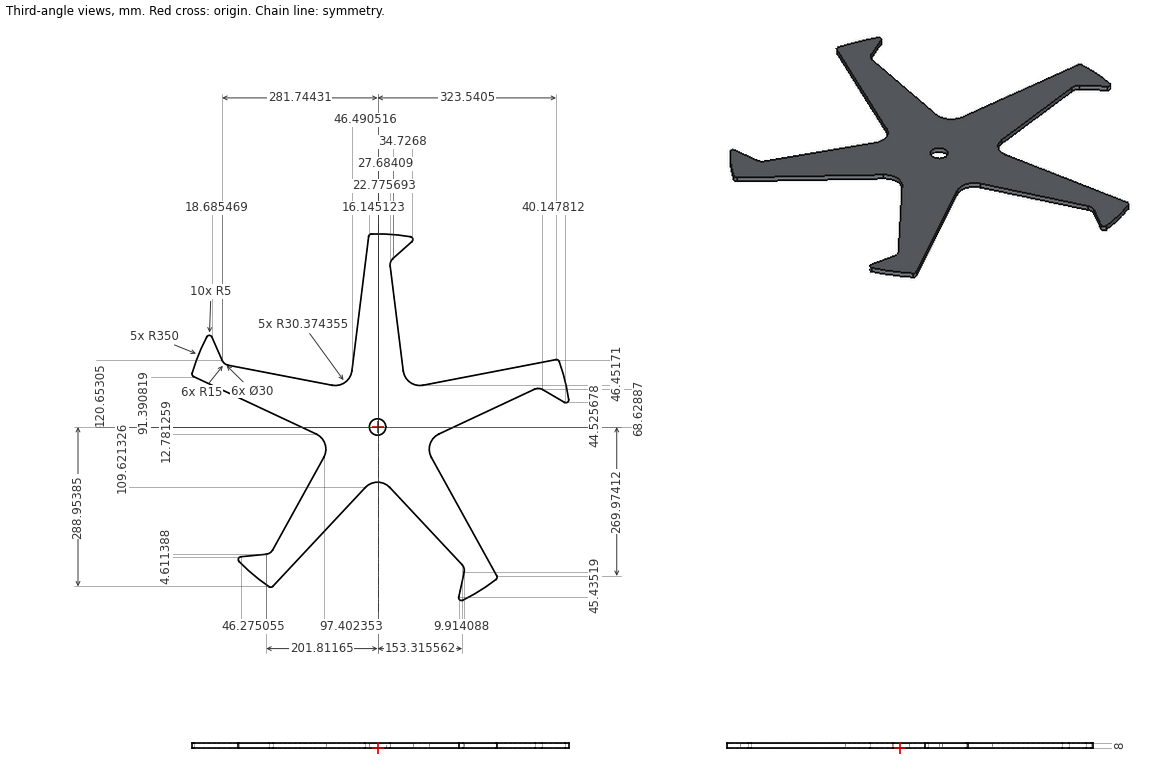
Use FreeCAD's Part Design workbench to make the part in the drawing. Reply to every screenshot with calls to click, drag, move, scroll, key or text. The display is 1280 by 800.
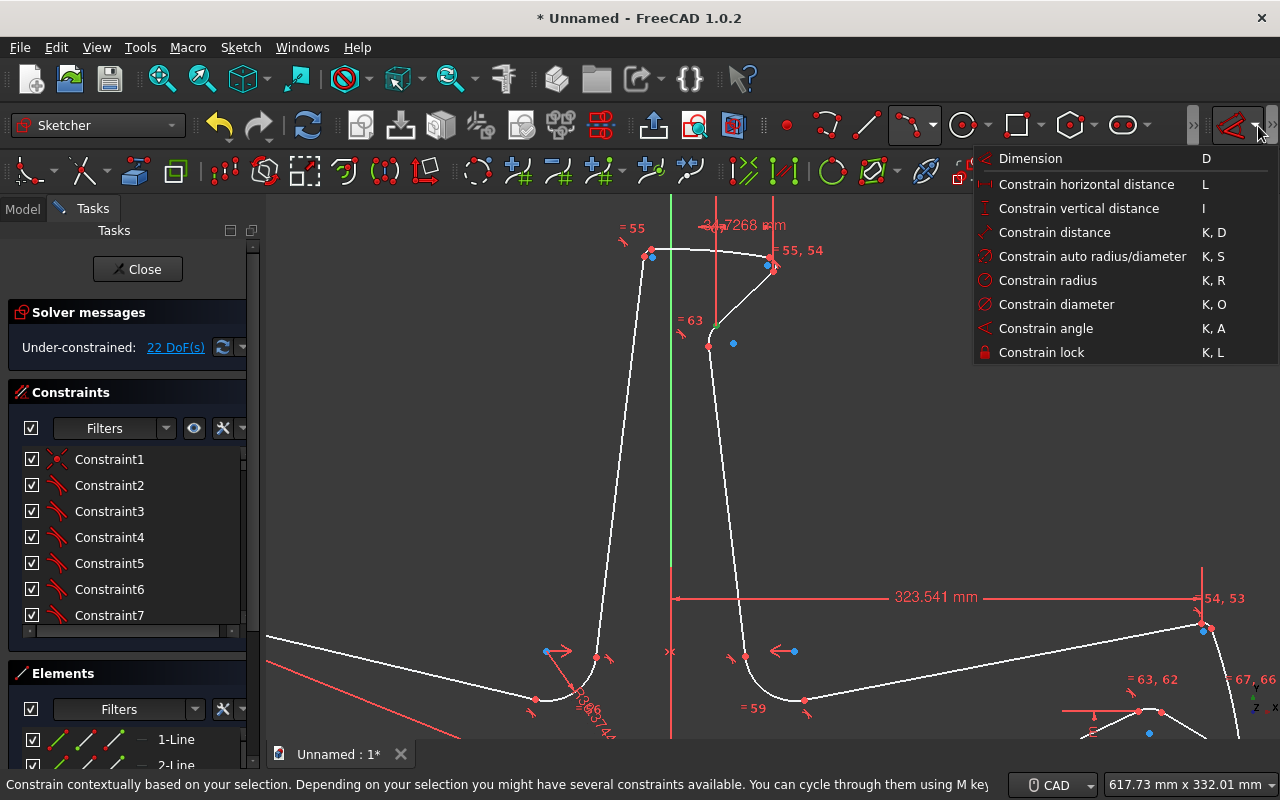
click(1126, 184)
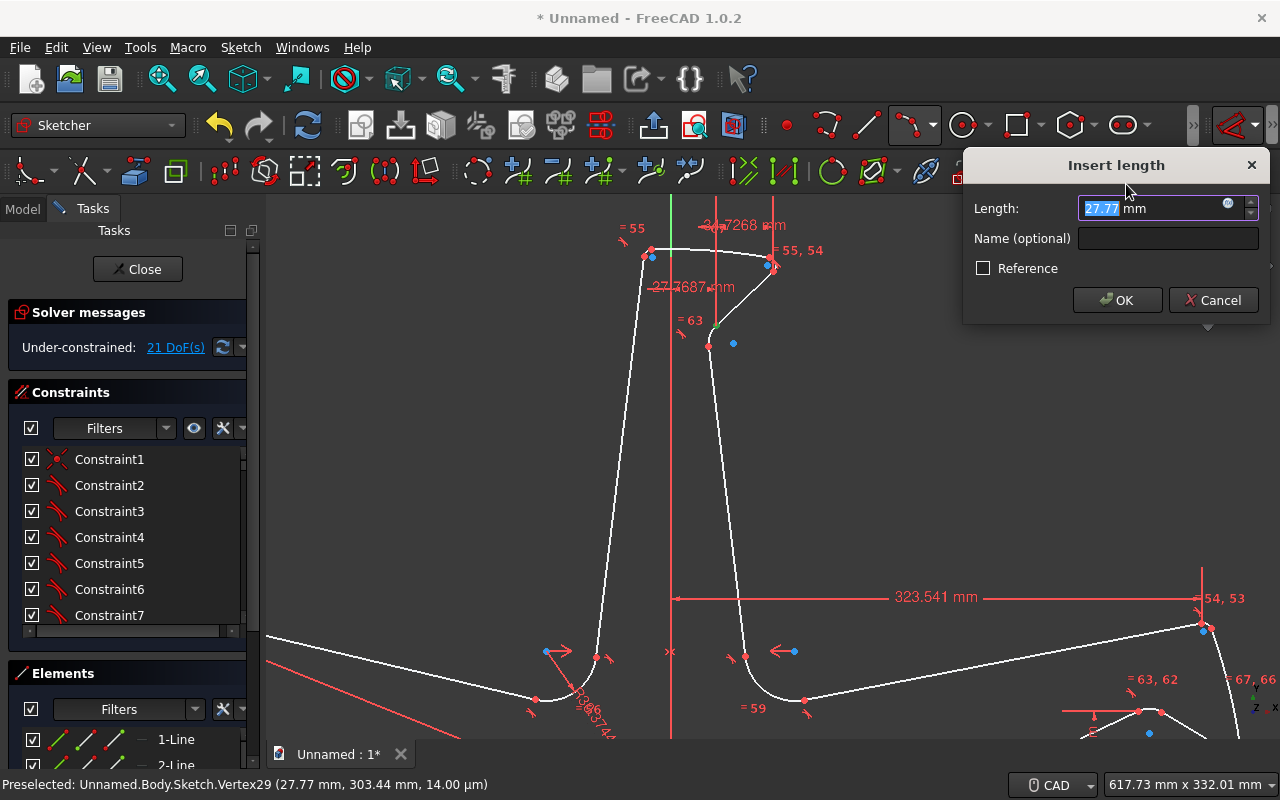
text(27.68409)
key(Return)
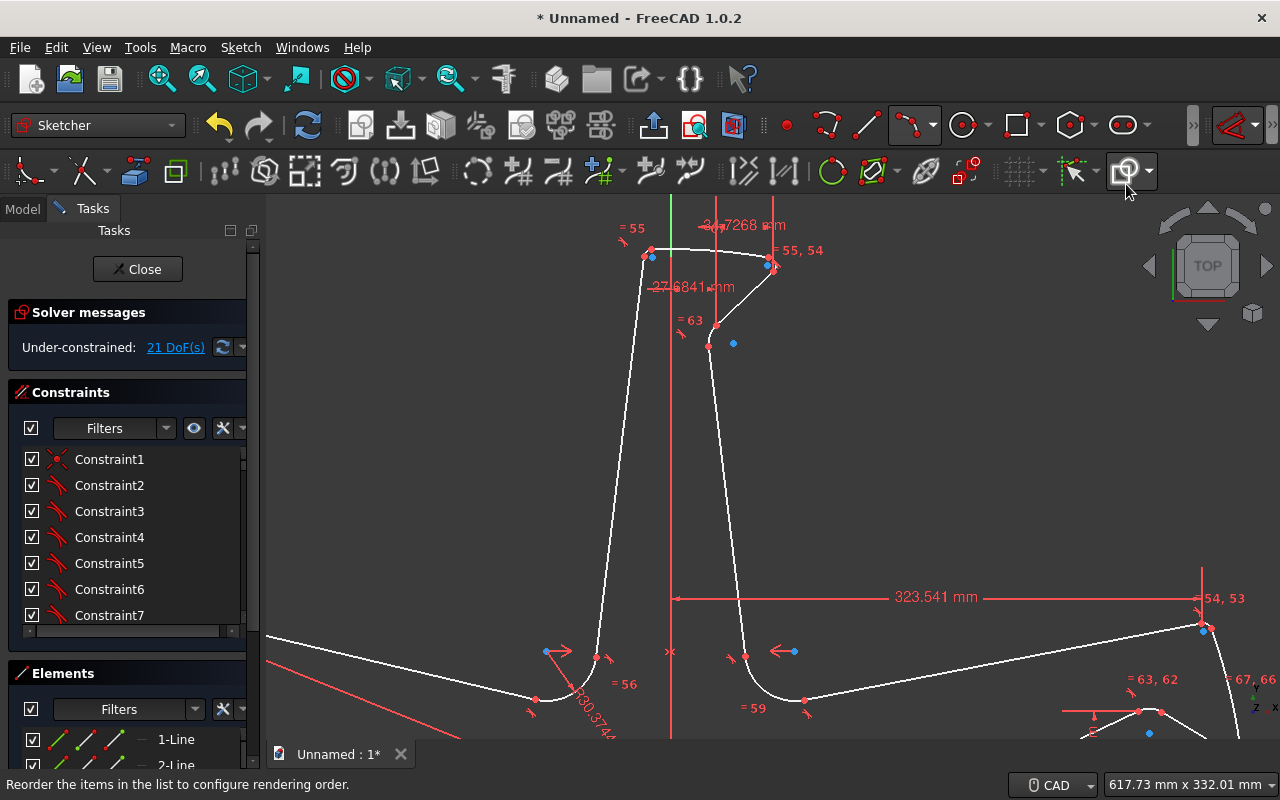
scroll(715, 325, down, 6)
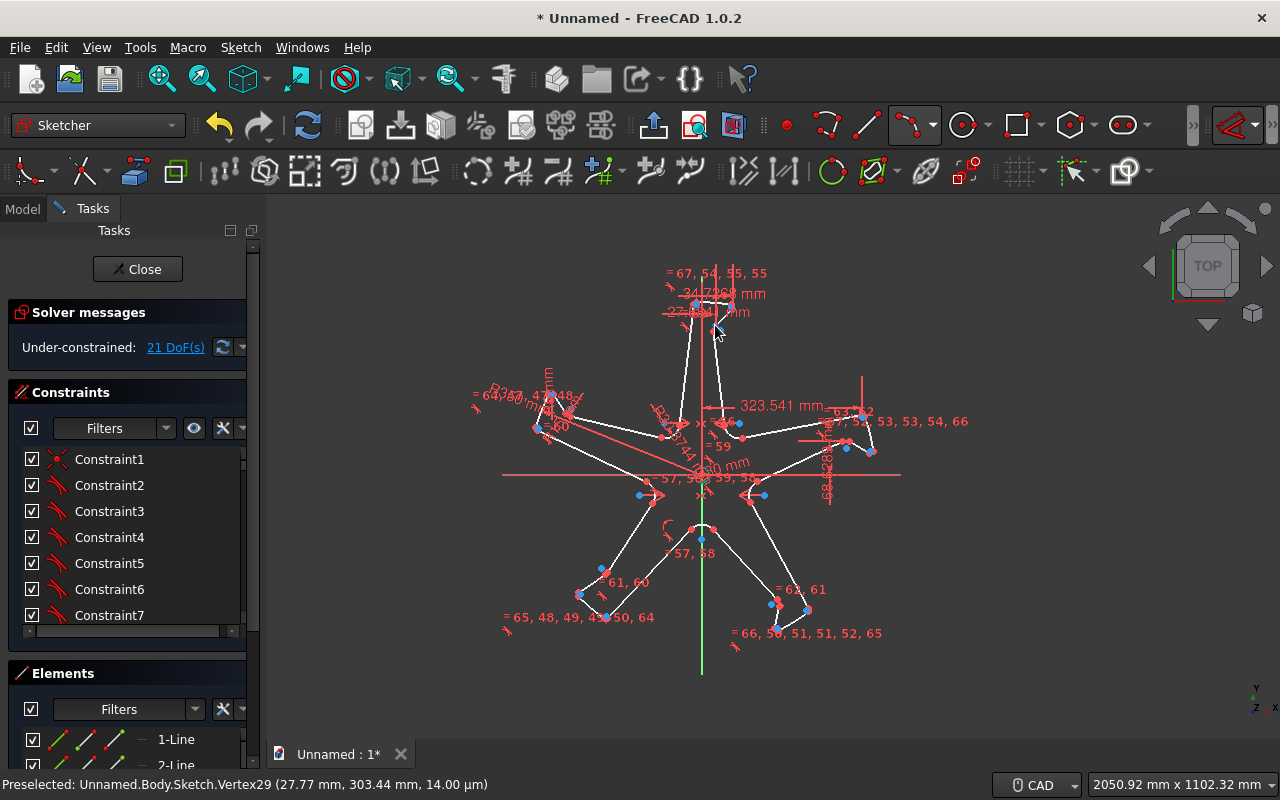
scroll(597, 580, up, 15)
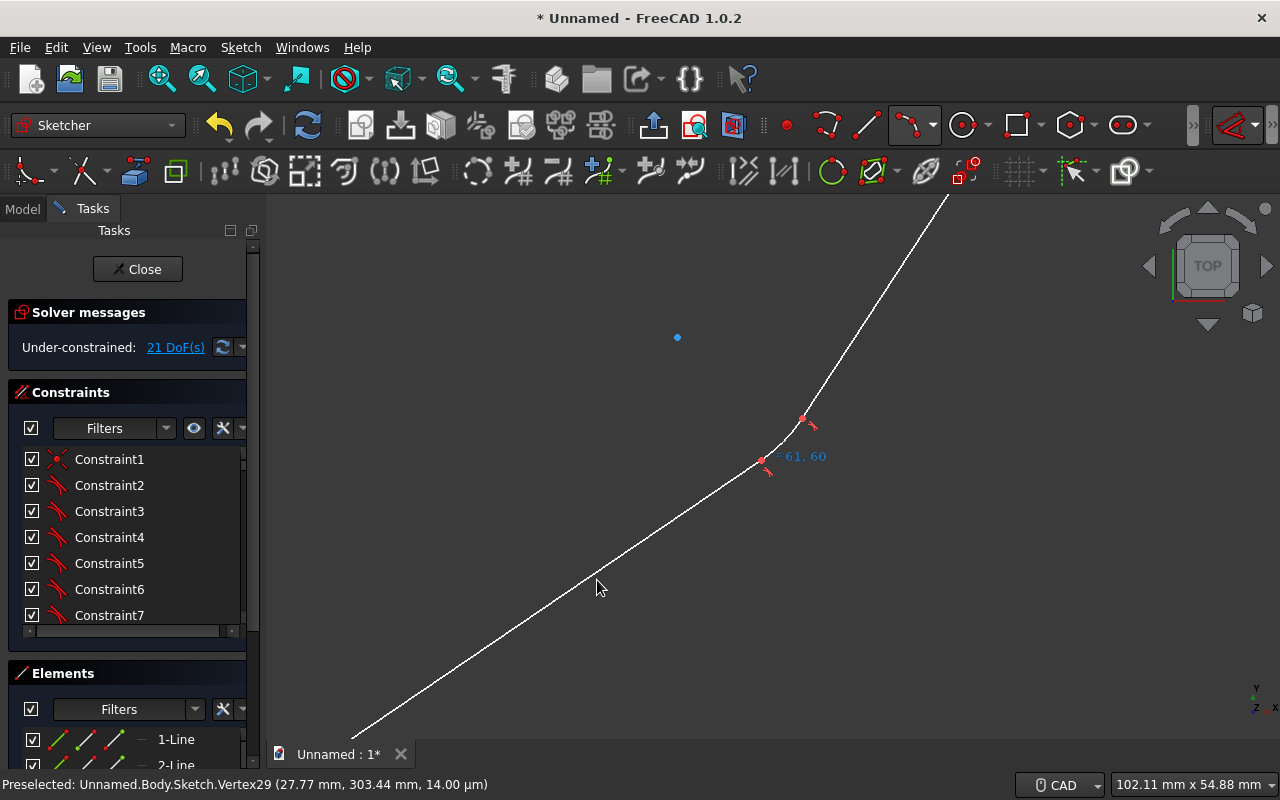
click(601, 569)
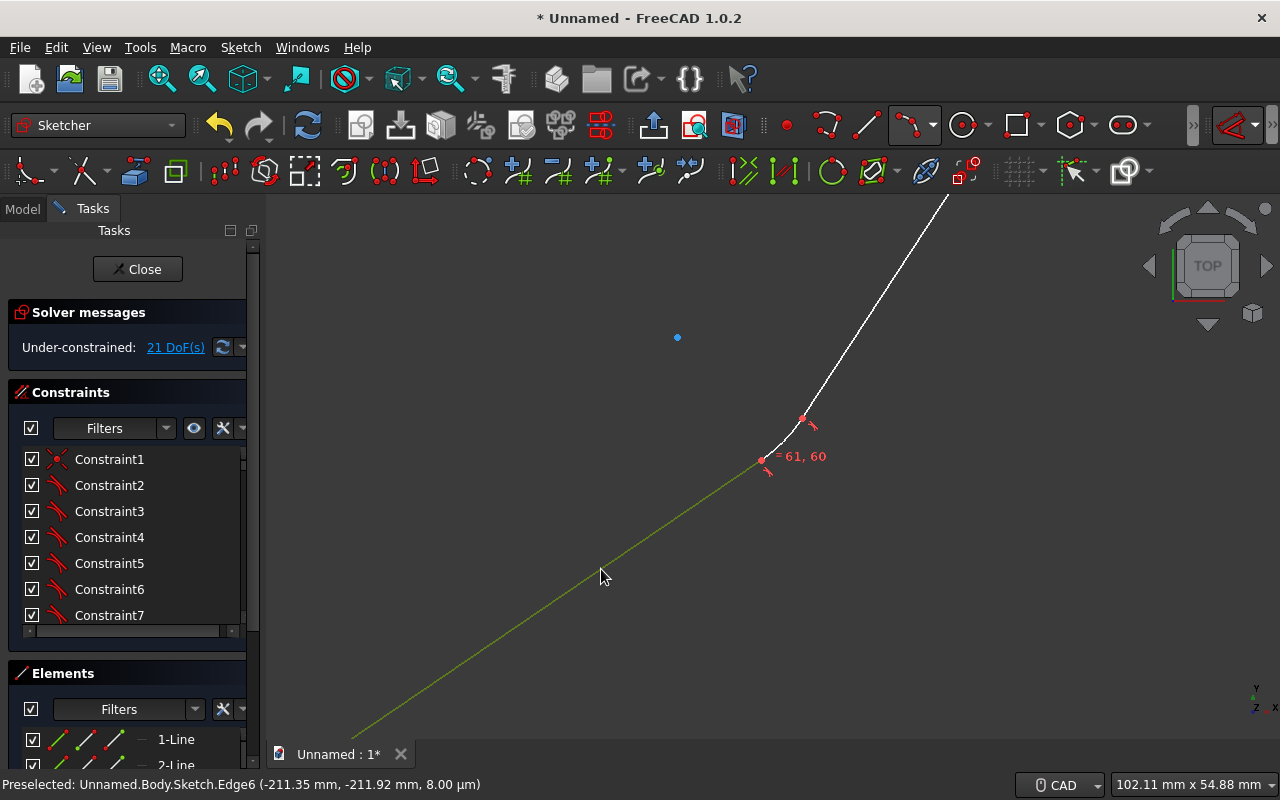
key(i)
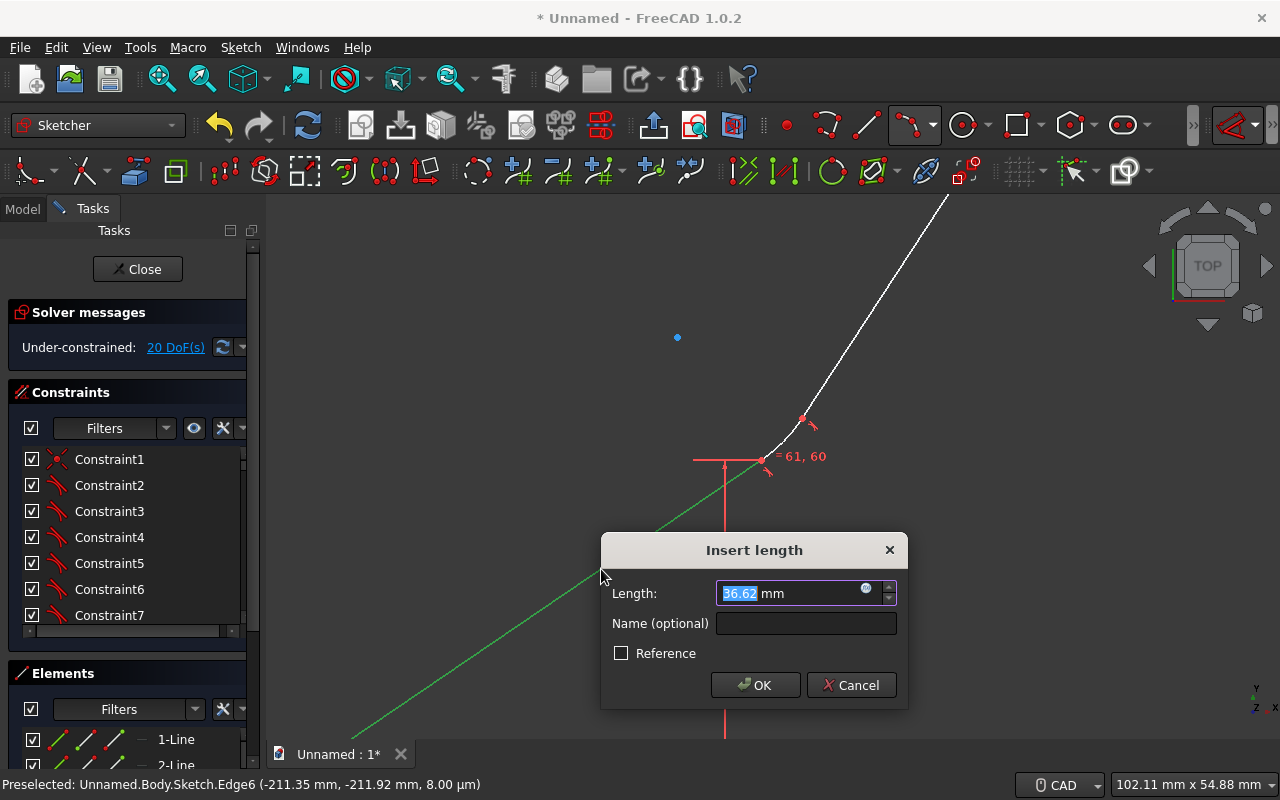
text(4.611388)
key(Return)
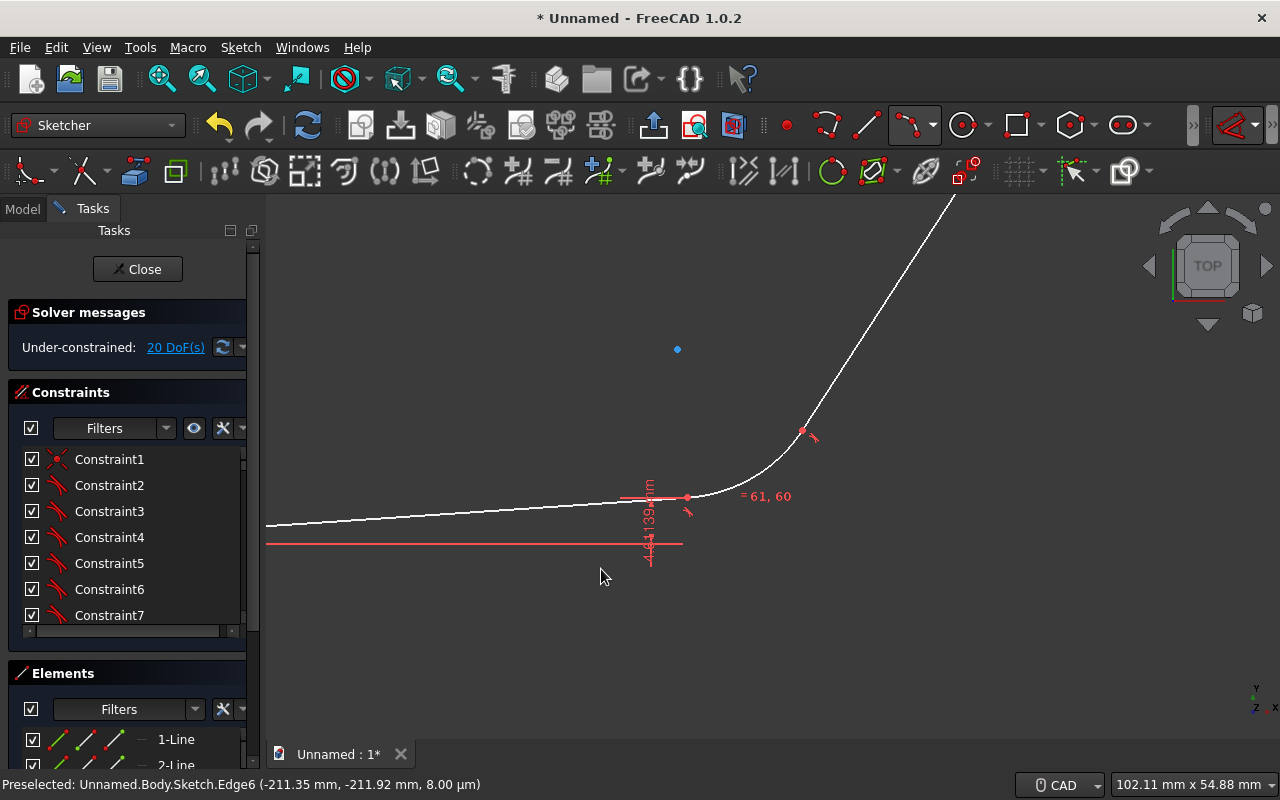
scroll(597, 581, down, 15)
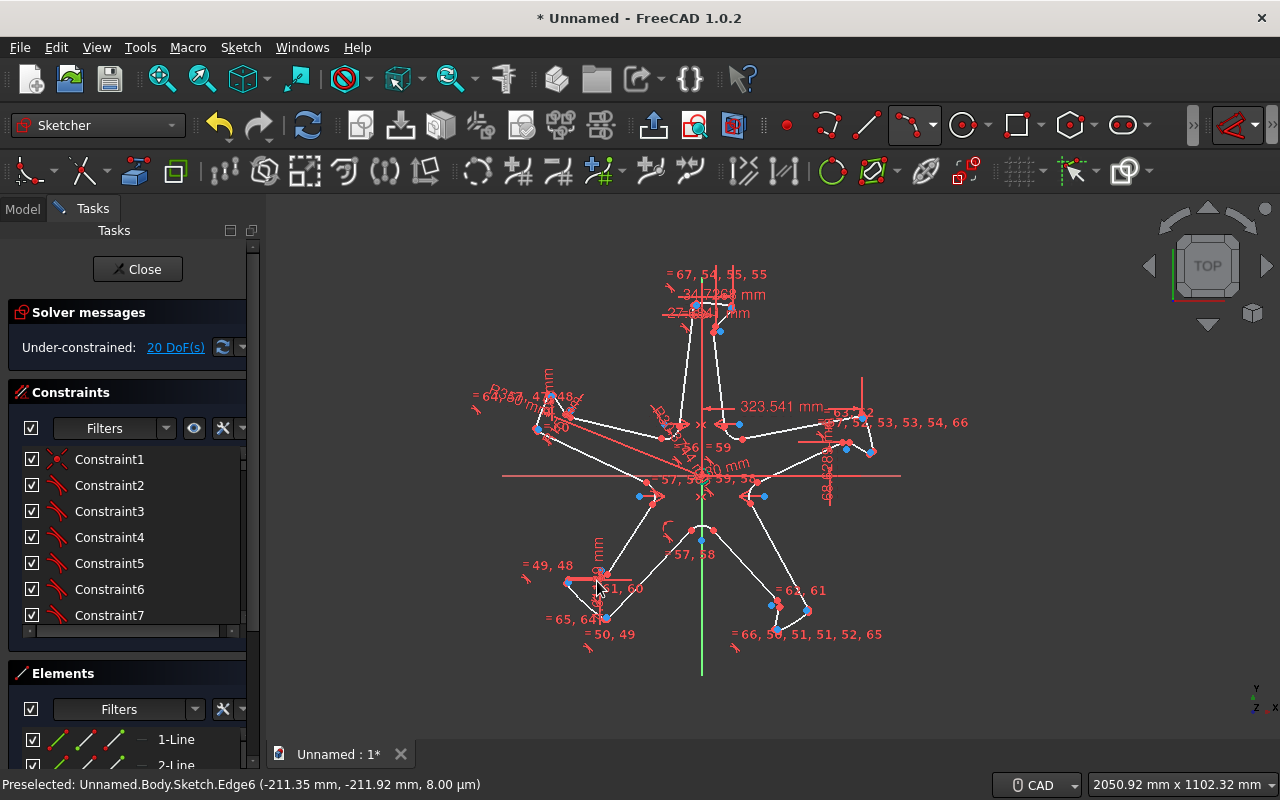
scroll(778, 614, up, 11)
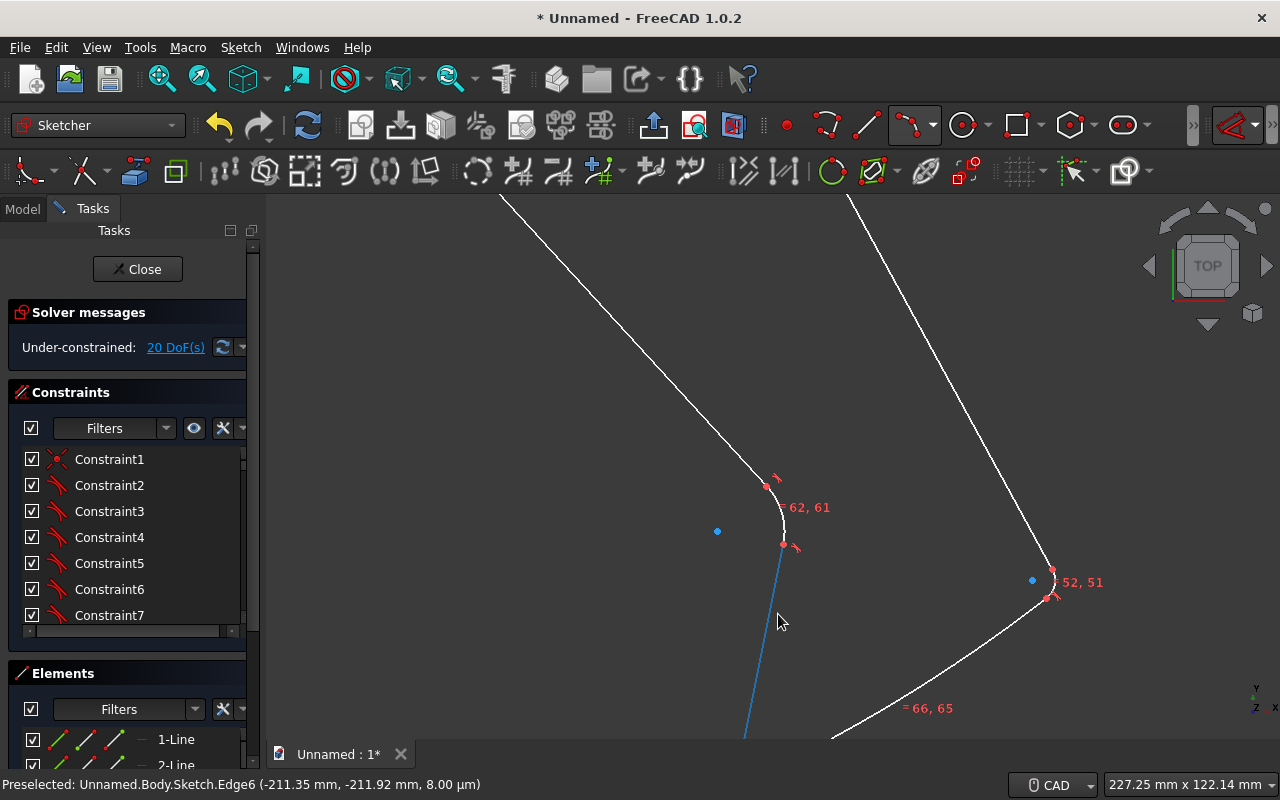
click(771, 604)